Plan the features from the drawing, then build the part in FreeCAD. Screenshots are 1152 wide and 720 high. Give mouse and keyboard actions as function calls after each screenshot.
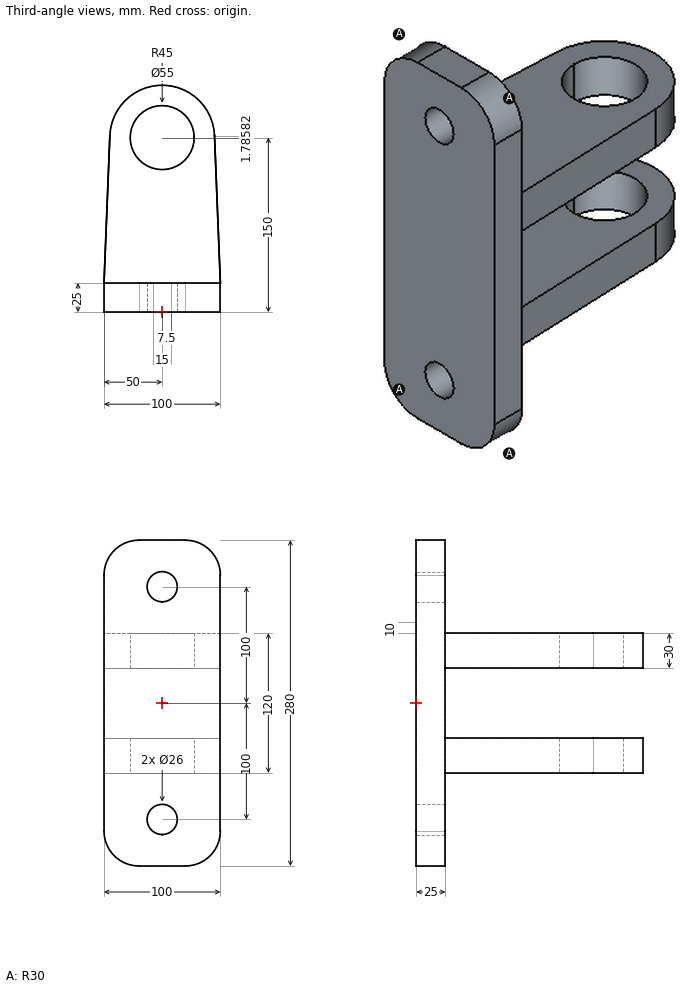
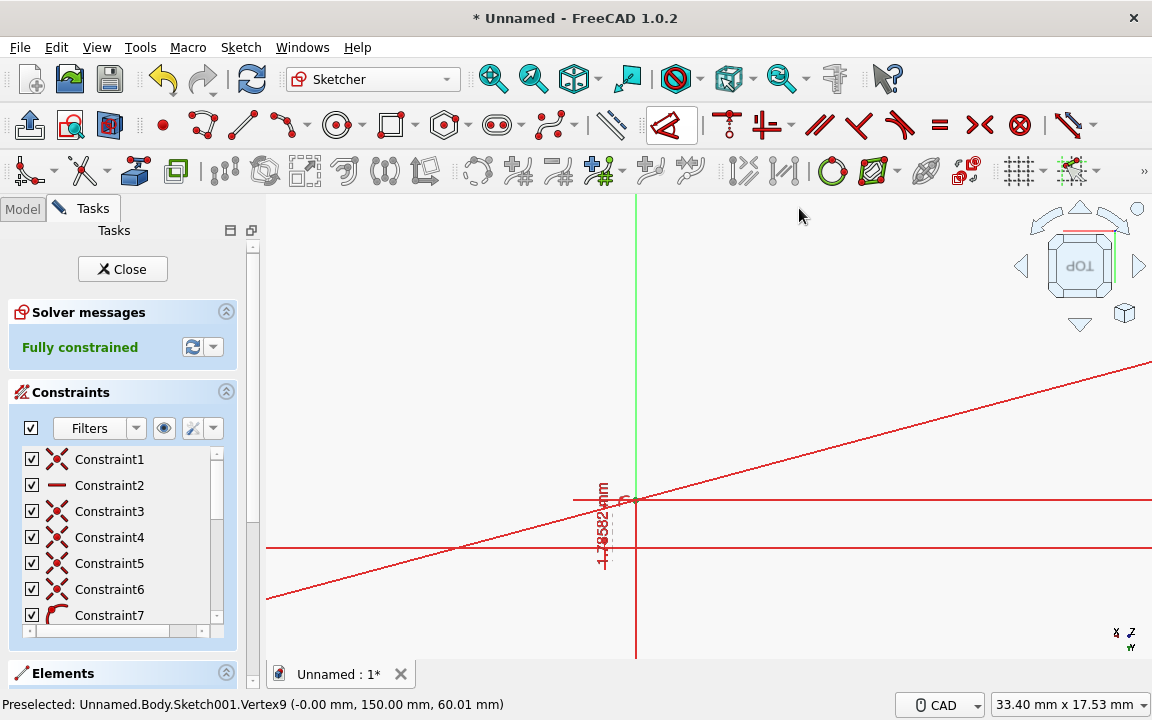
click(123, 269)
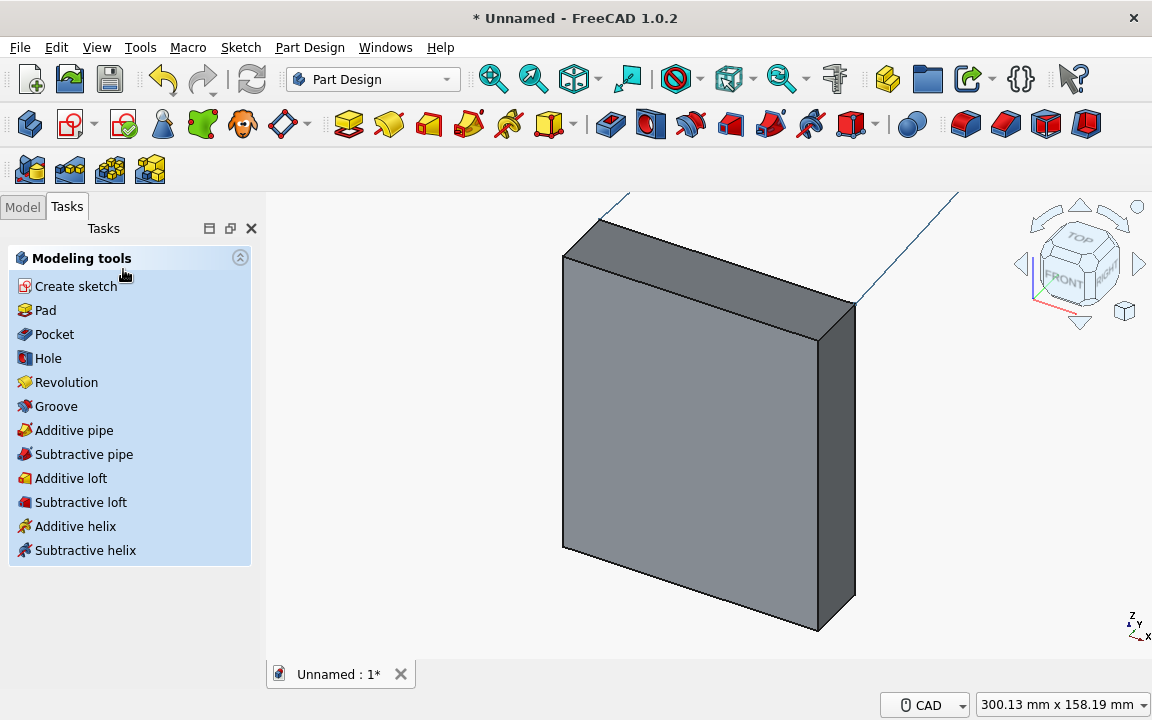
click(350, 124)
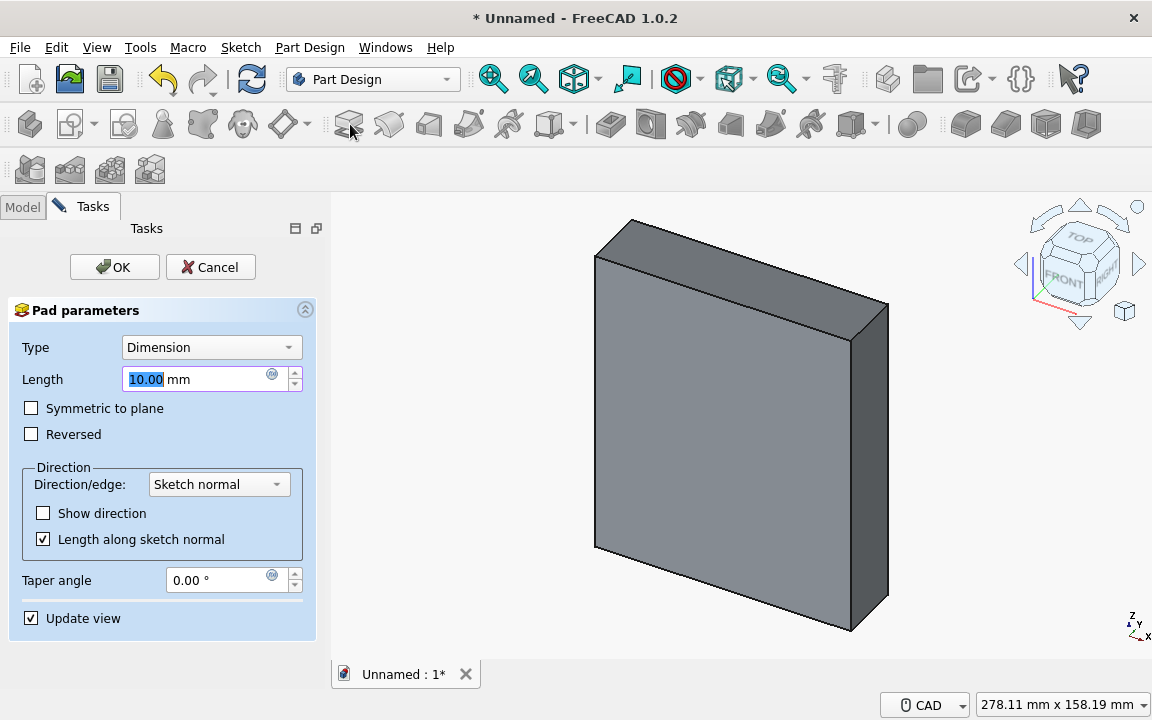
text(30)
key(Tab)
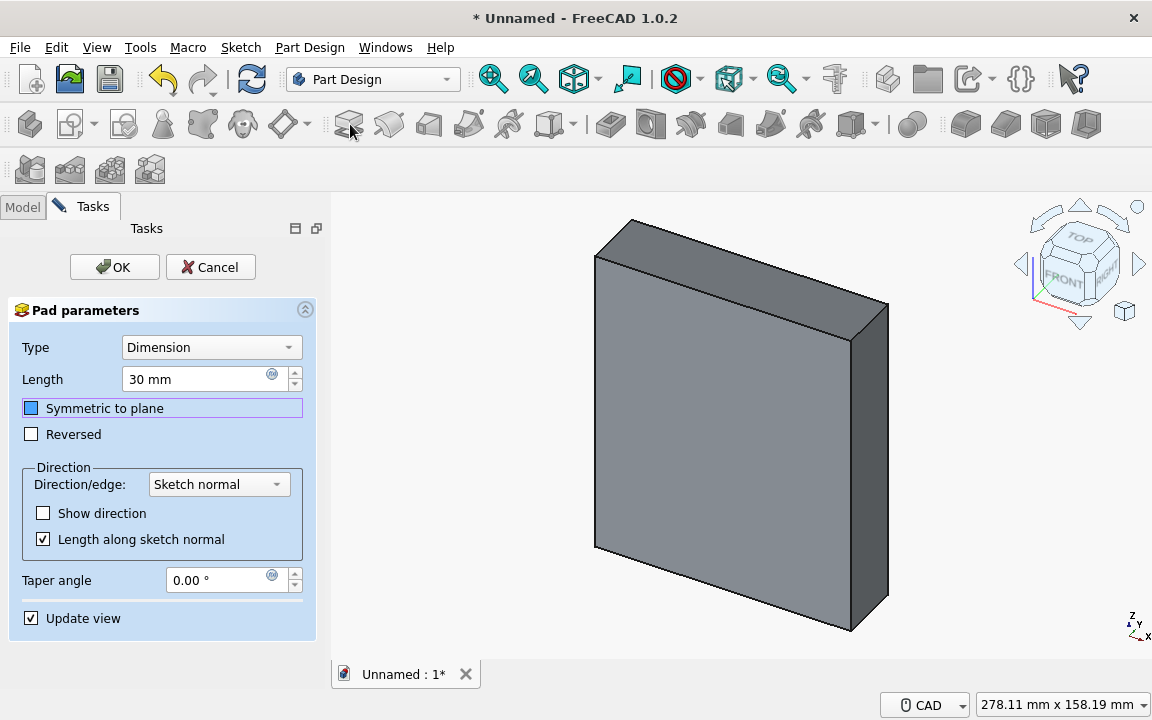
click(30, 434)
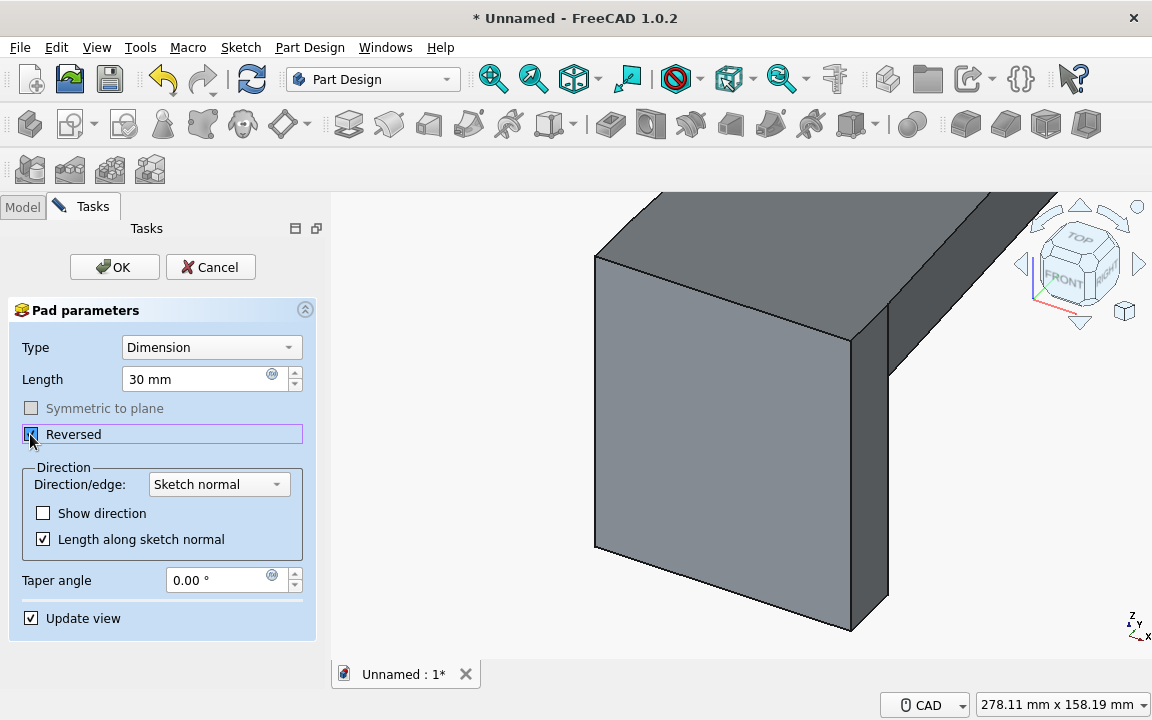
click(115, 267)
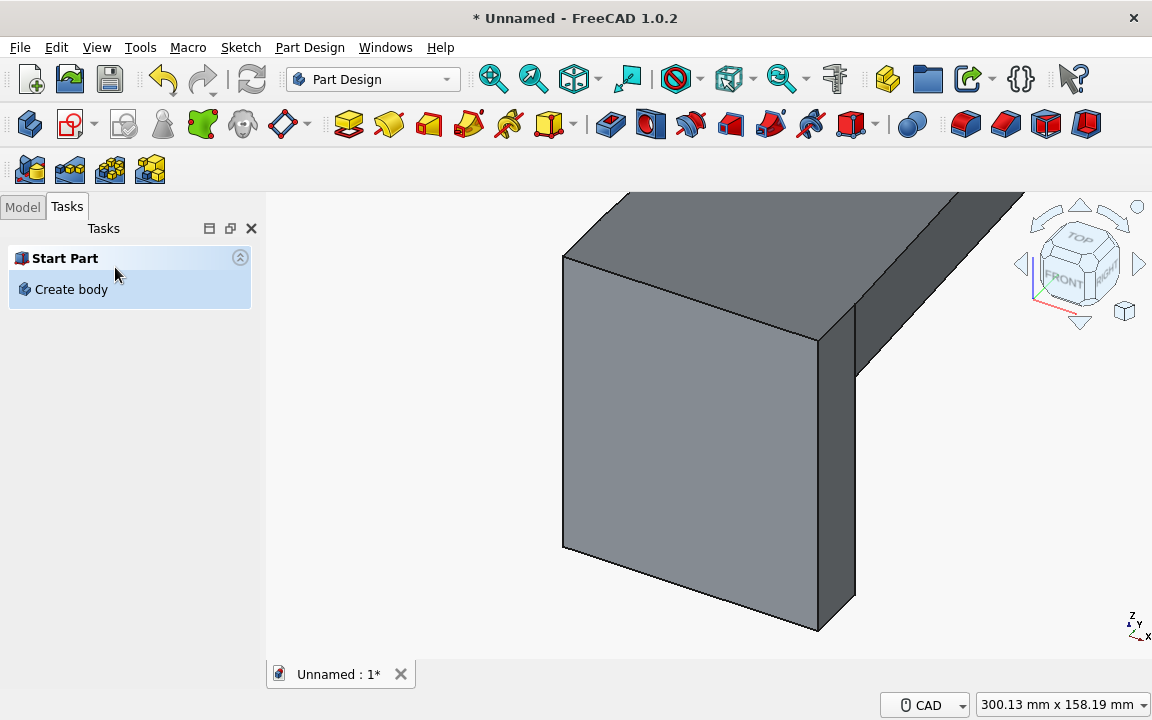
click(494, 80)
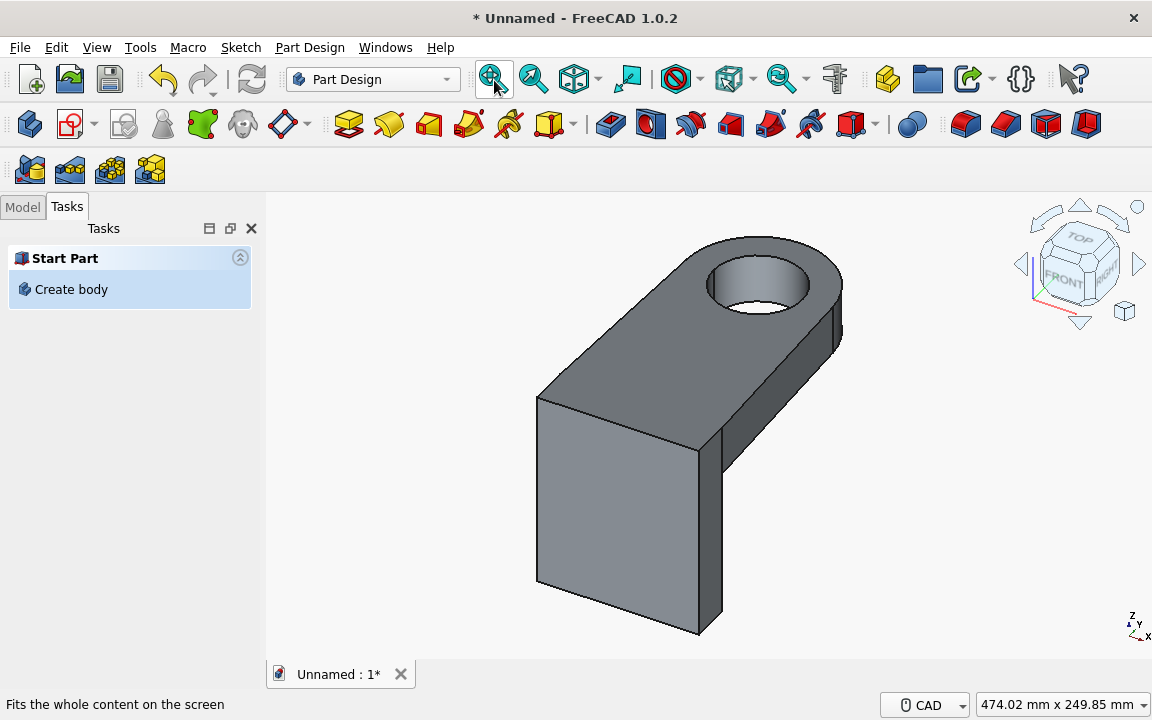
click(683, 358)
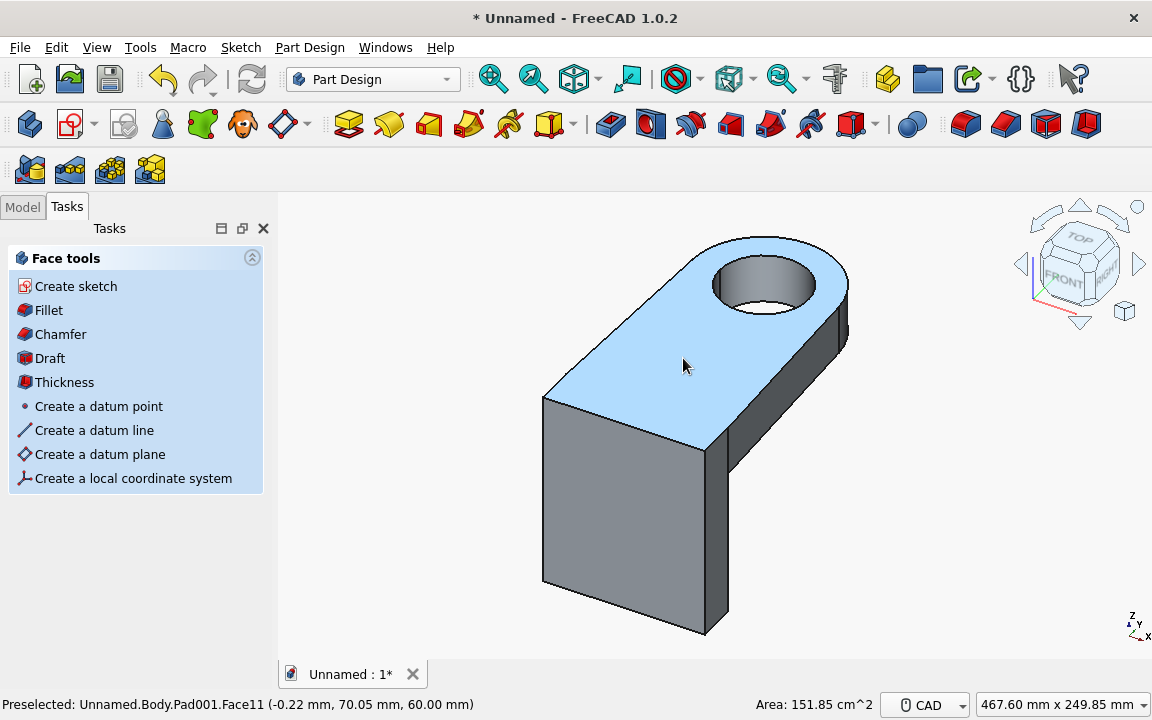
click(70, 124)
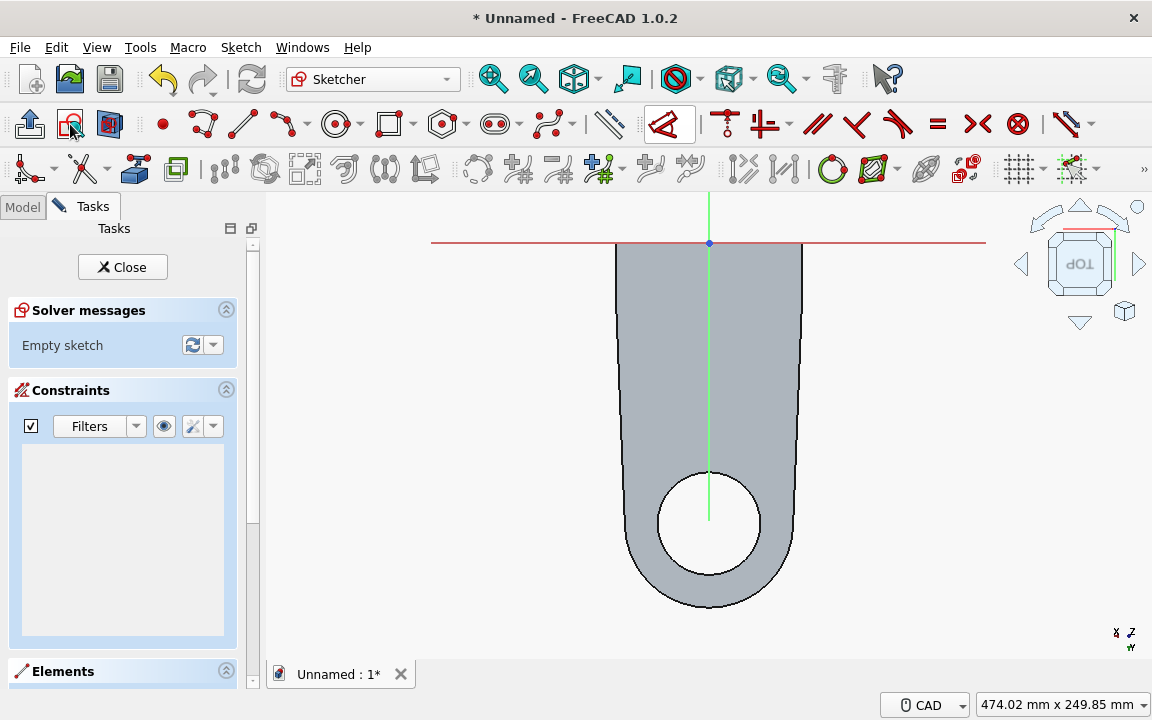
scroll(723, 235, up, 9)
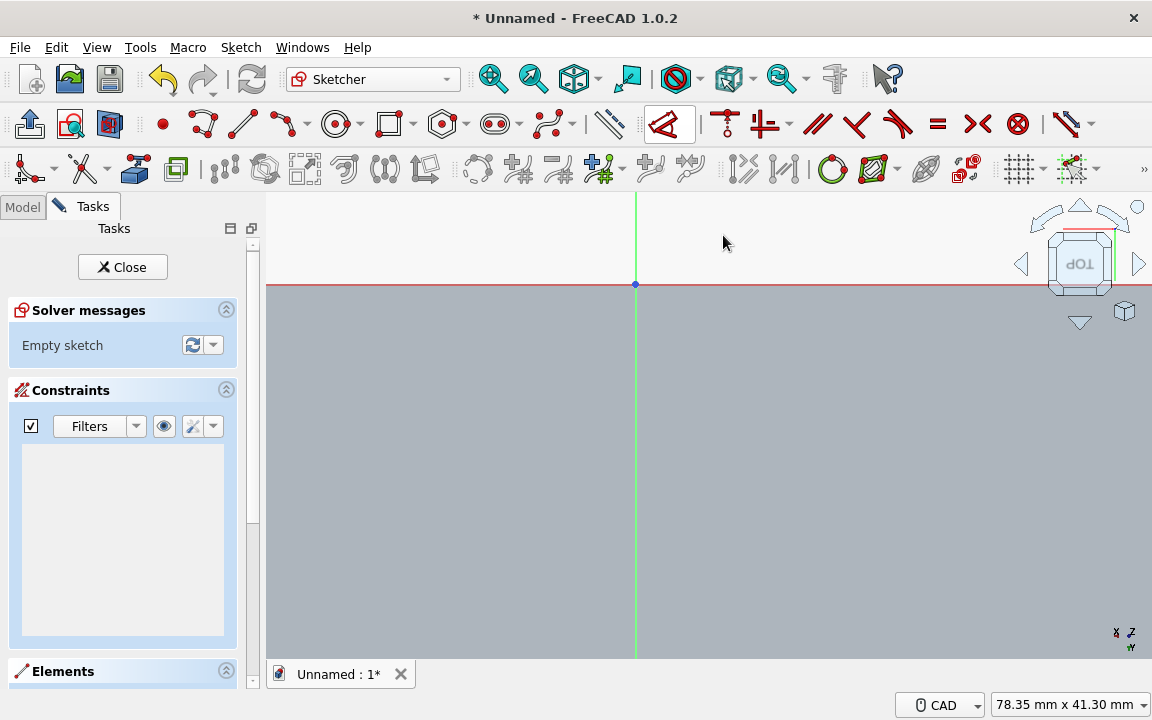
click(390, 124)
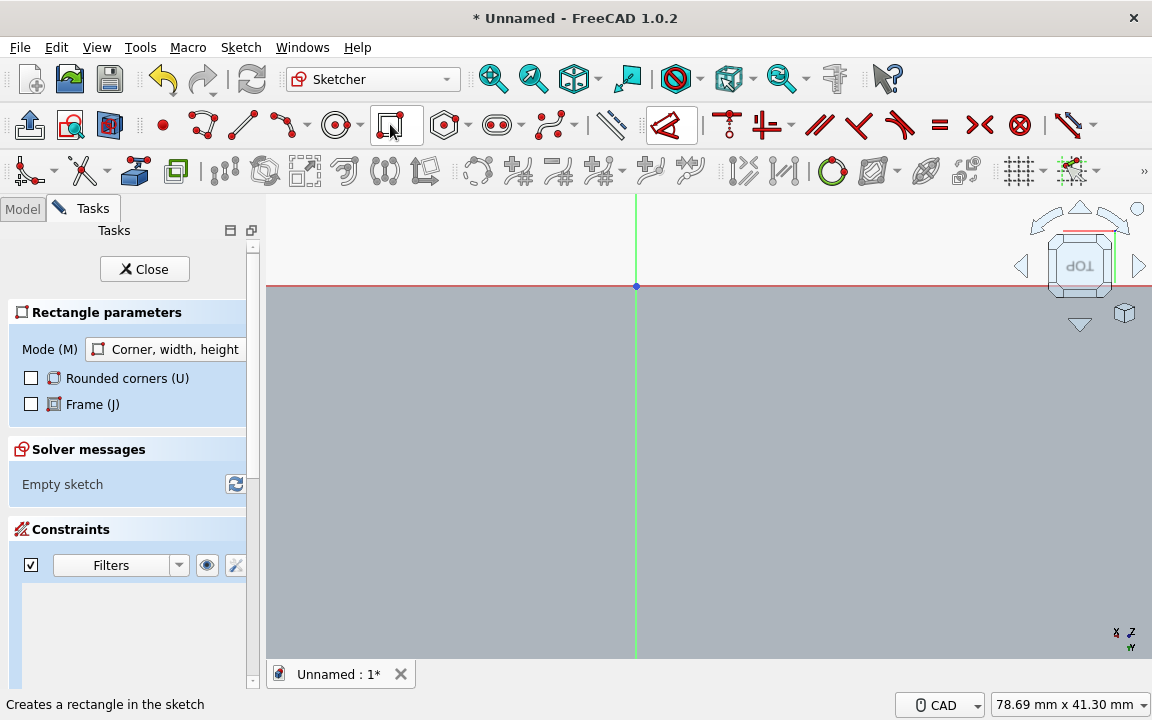
click(552, 286)
click(720, 568)
key(Escape)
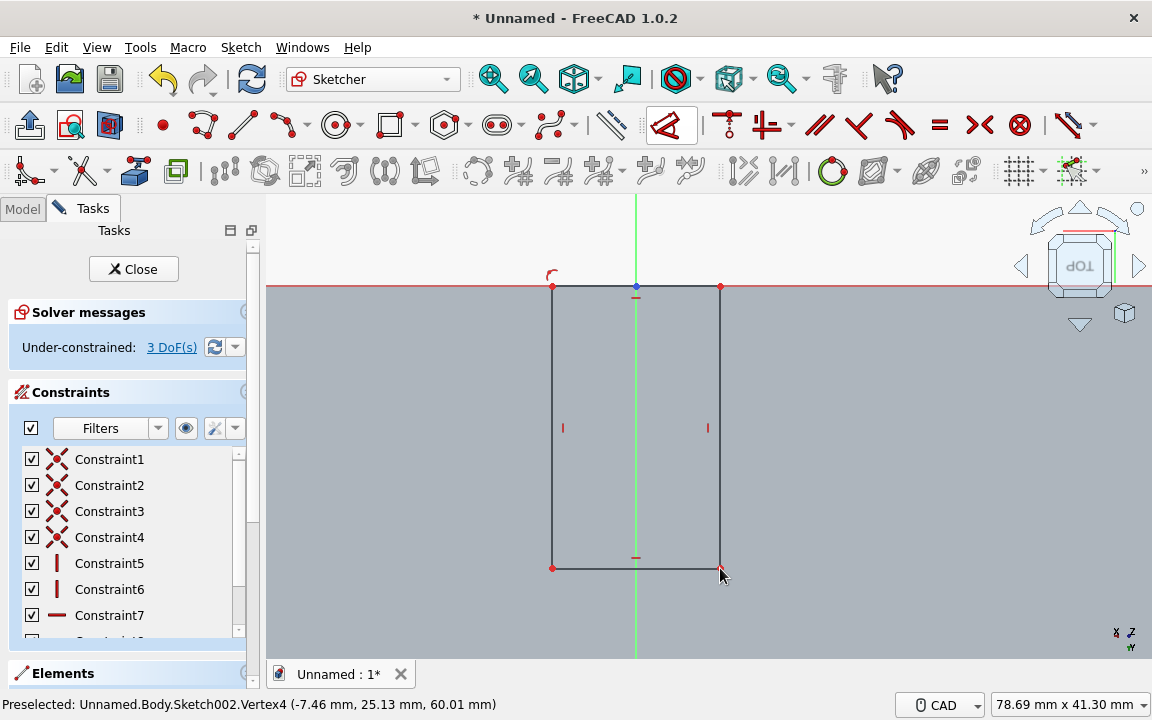
click(552, 371)